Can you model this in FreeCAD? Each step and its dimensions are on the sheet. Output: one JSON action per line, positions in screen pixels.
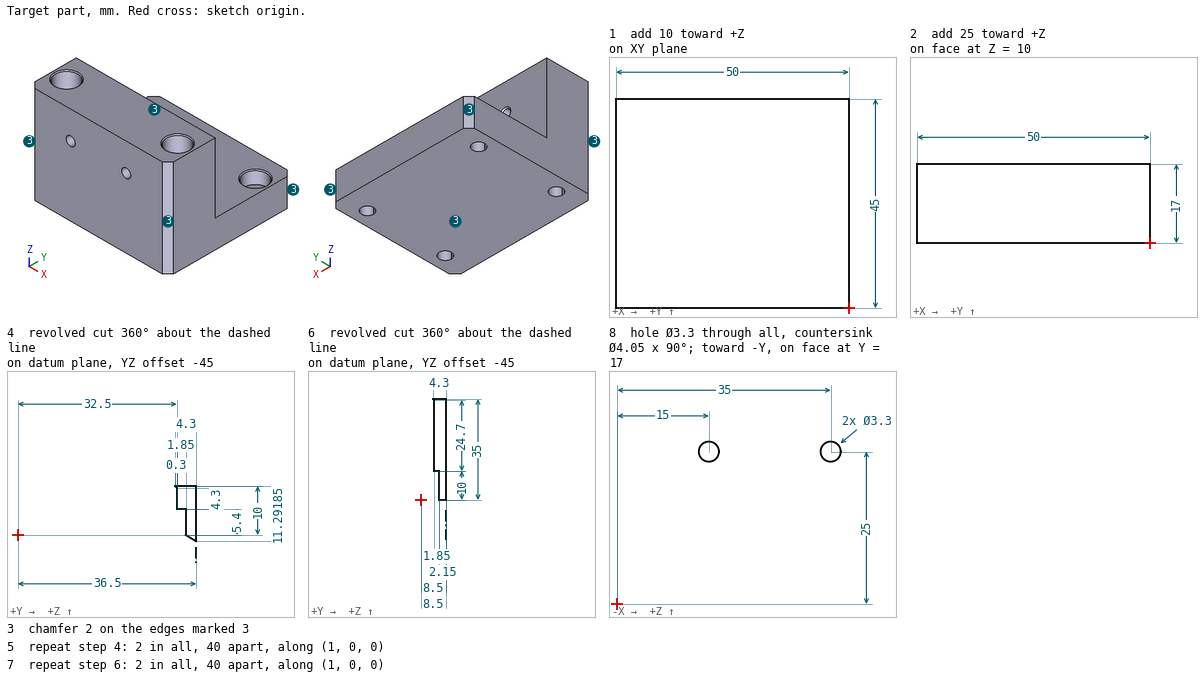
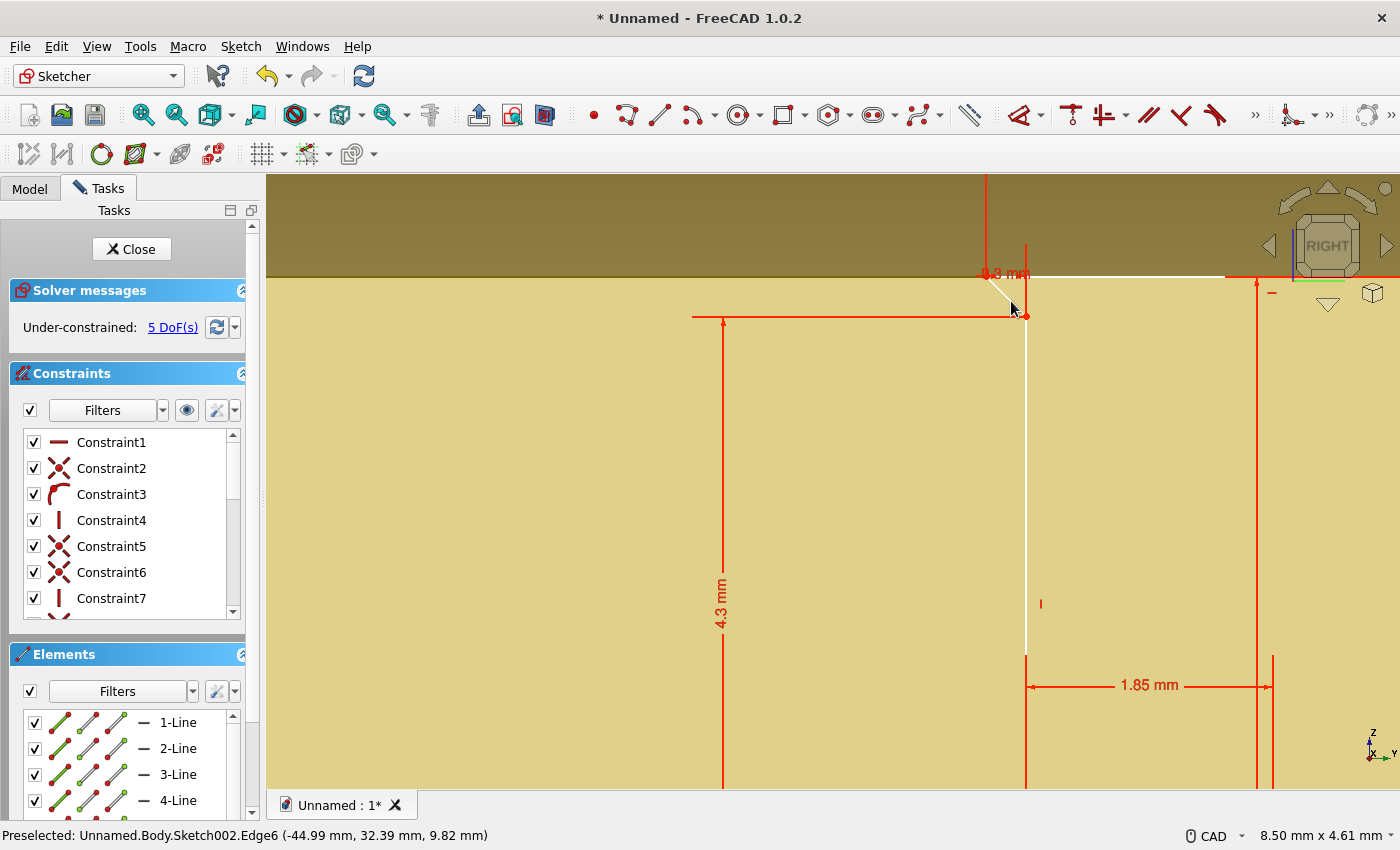
{"action": "scroll", "coordinate": [1021, 349], "scroll_direction": "down", "scroll_amount": 10}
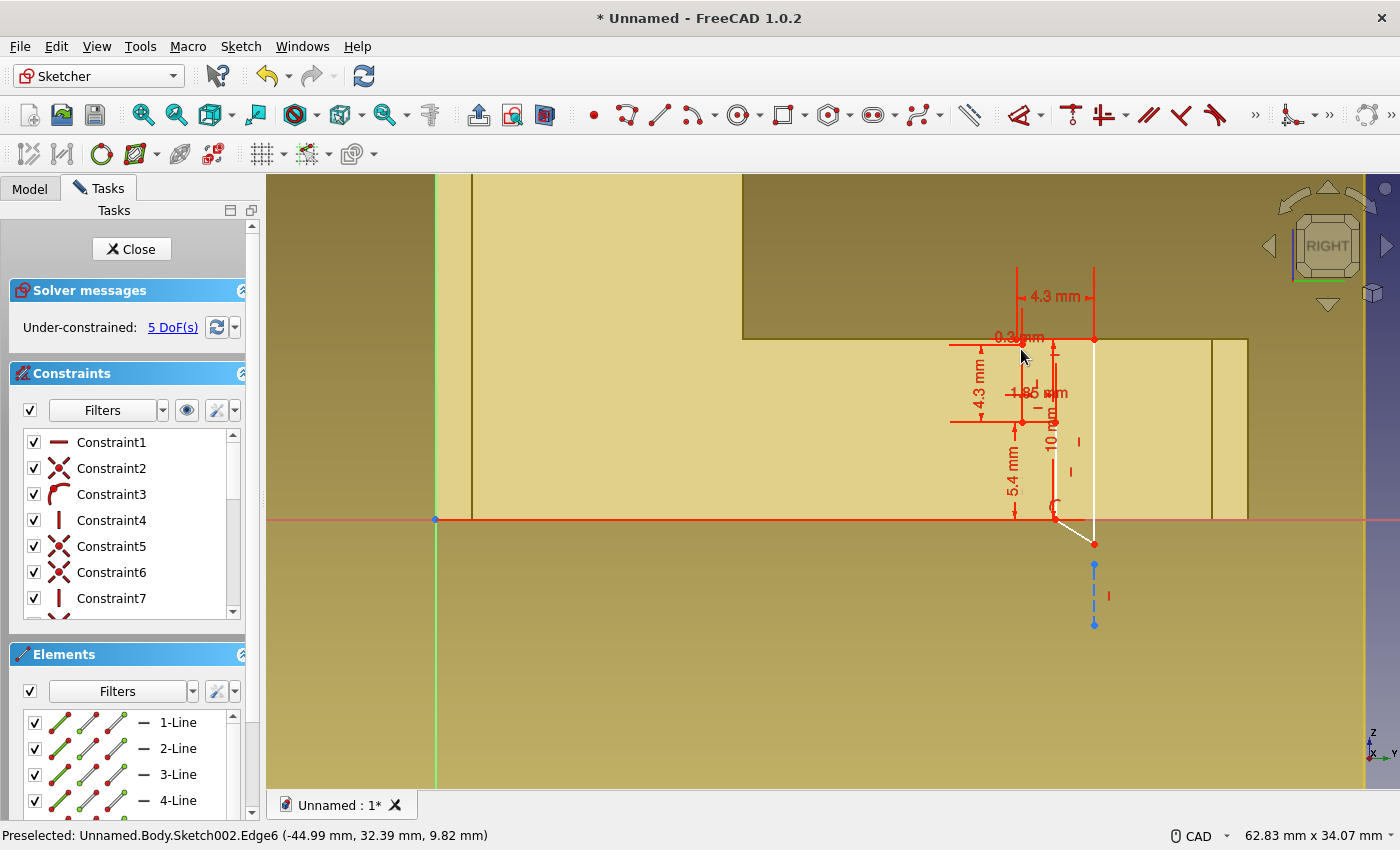
{"action": "left_click", "coordinate": [1022, 422]}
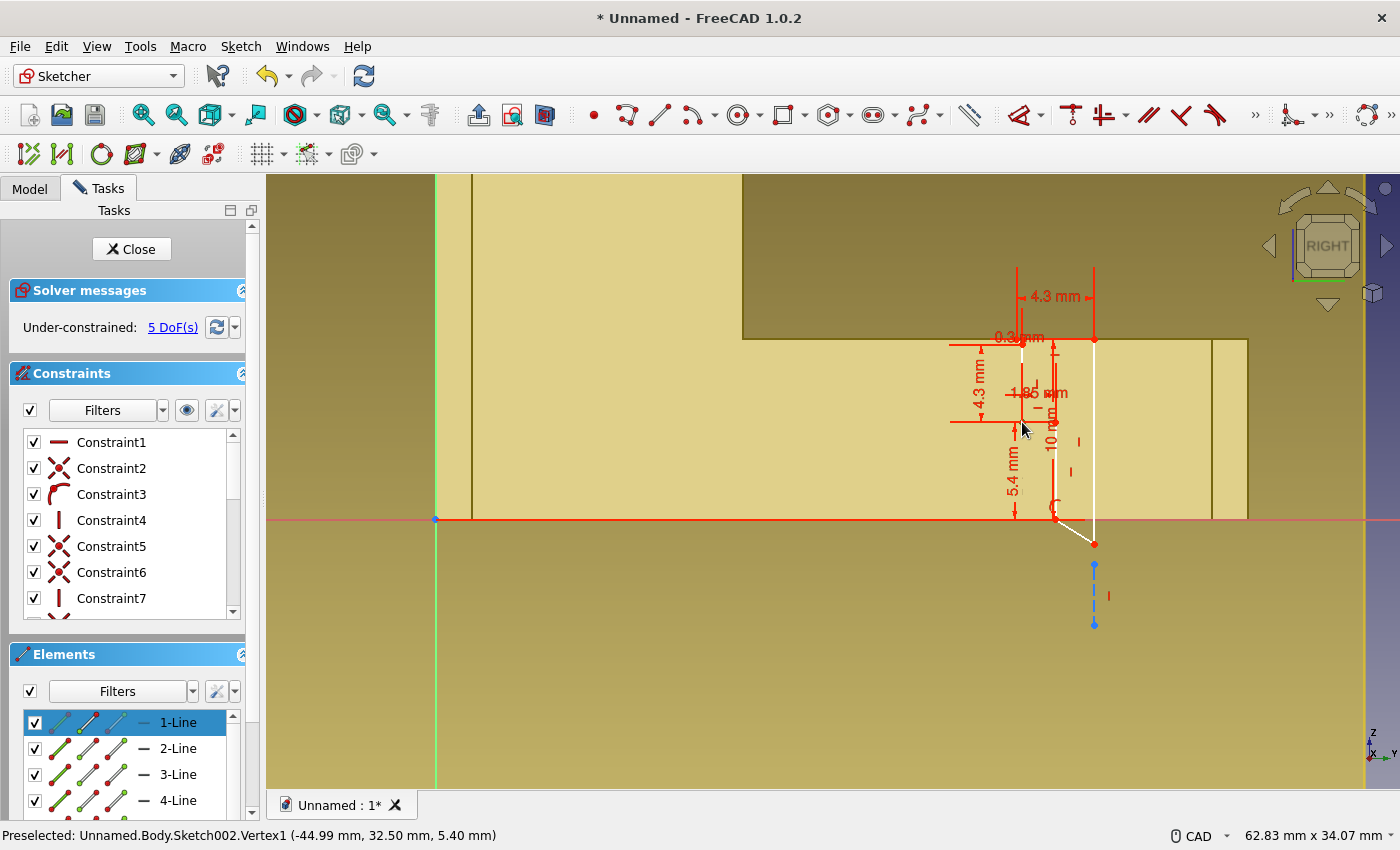
{"action": "key", "text": "l"}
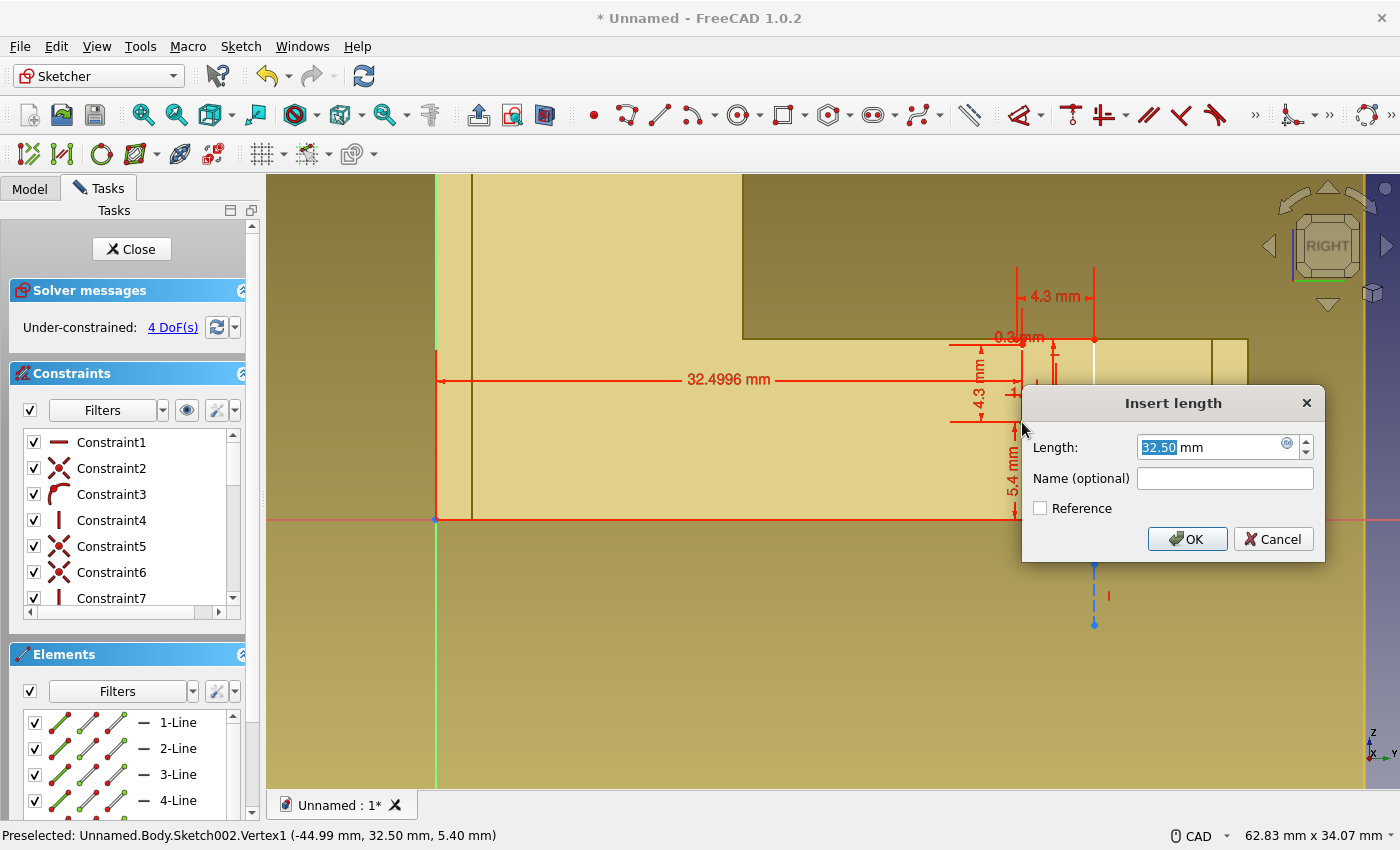
{"action": "type", "text": "32.5"}
{"action": "key", "text": "Return"}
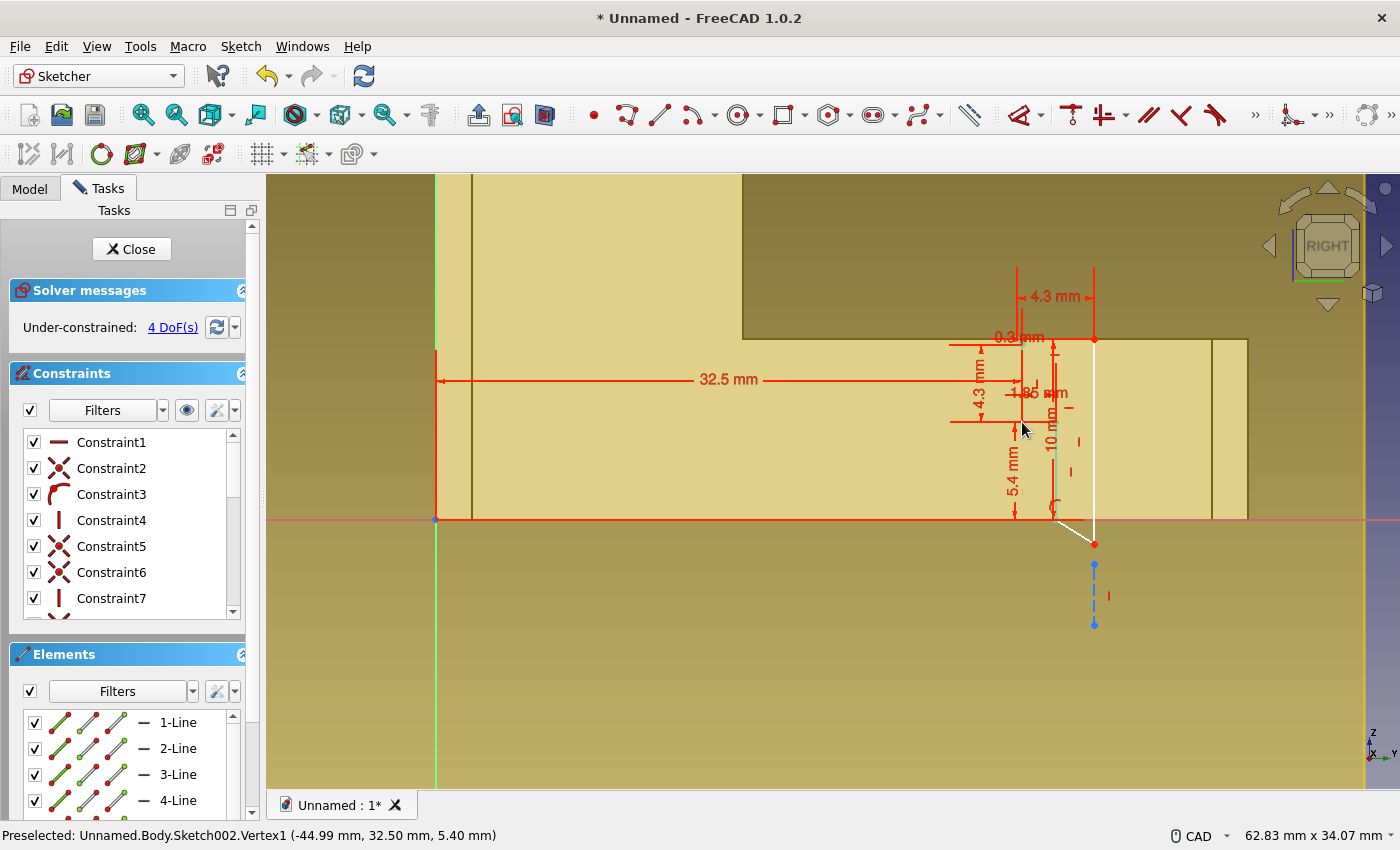
{"action": "left_click", "coordinate": [1094, 565]}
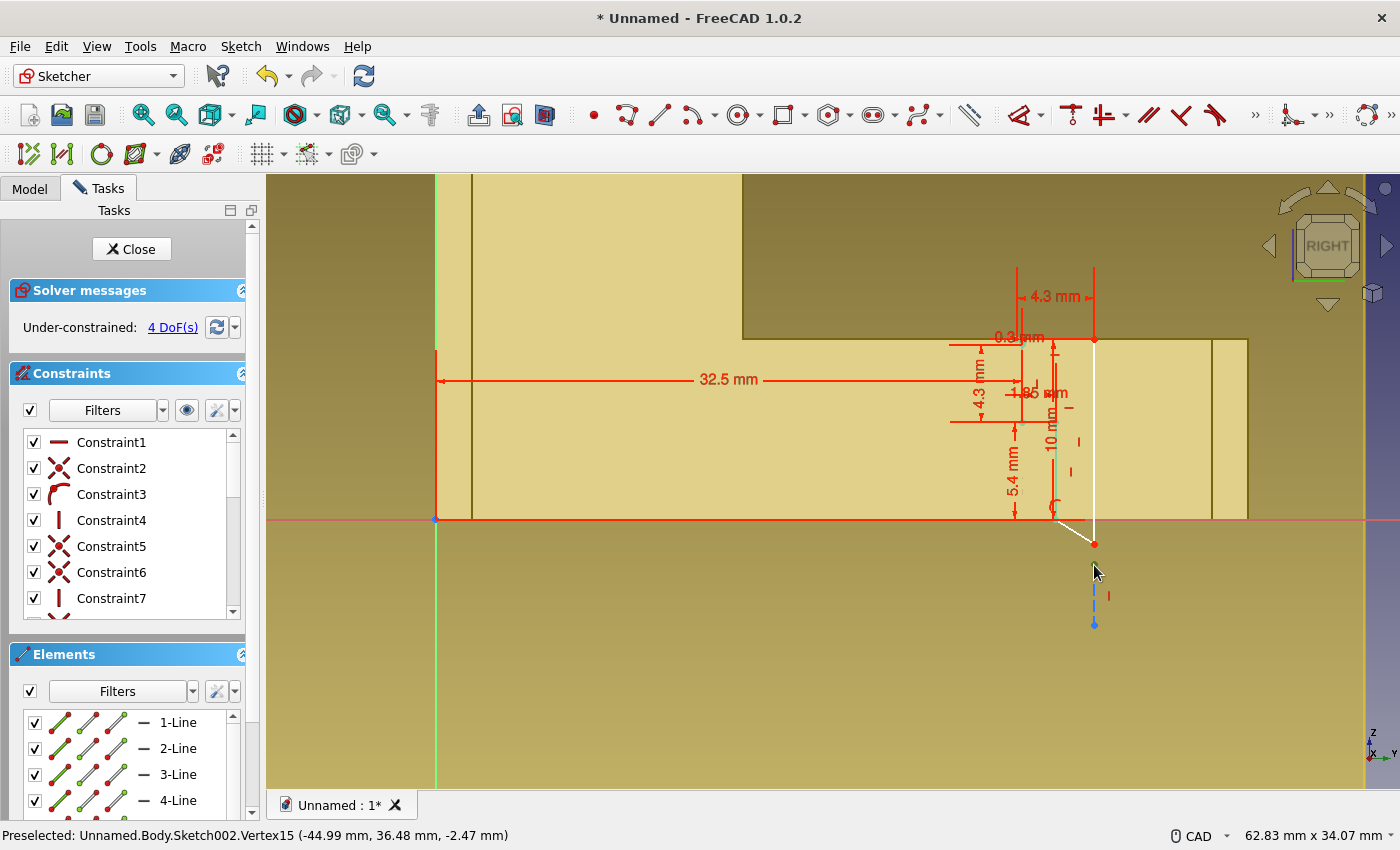
{"action": "key", "text": "l"}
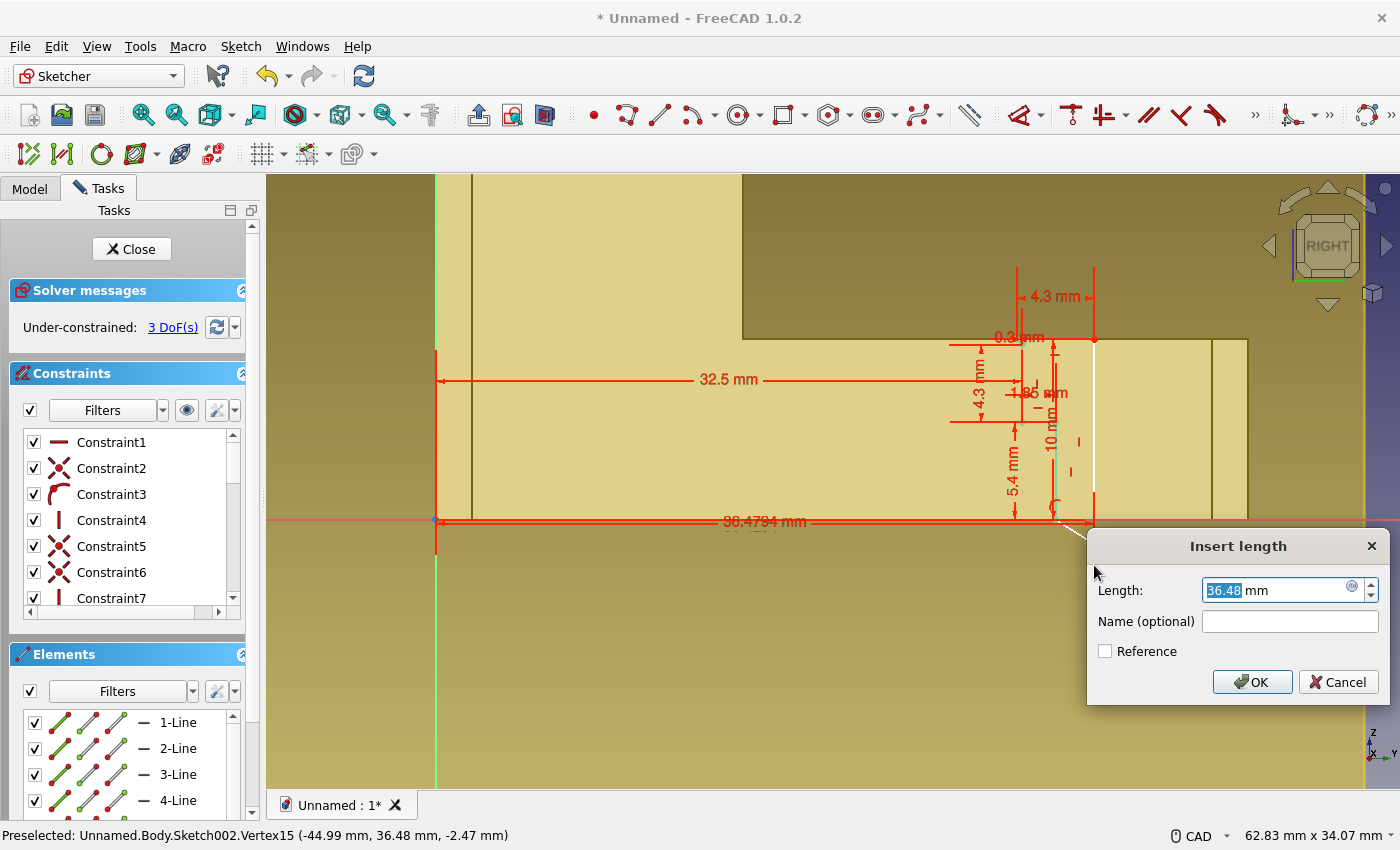
{"action": "type", "text": "36.5"}
{"action": "key", "text": "Return"}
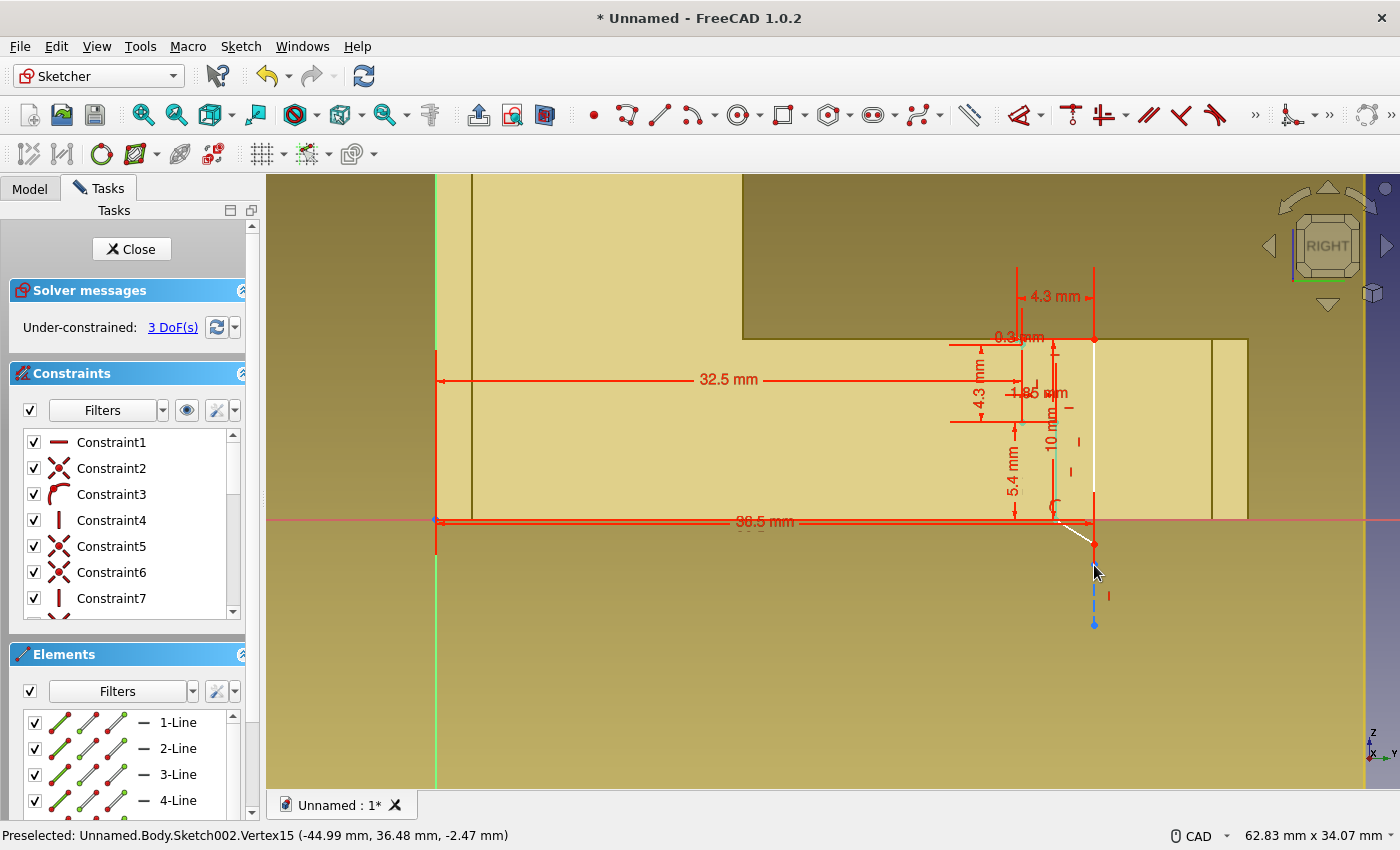
{"action": "left_click", "coordinate": [1094, 483]}